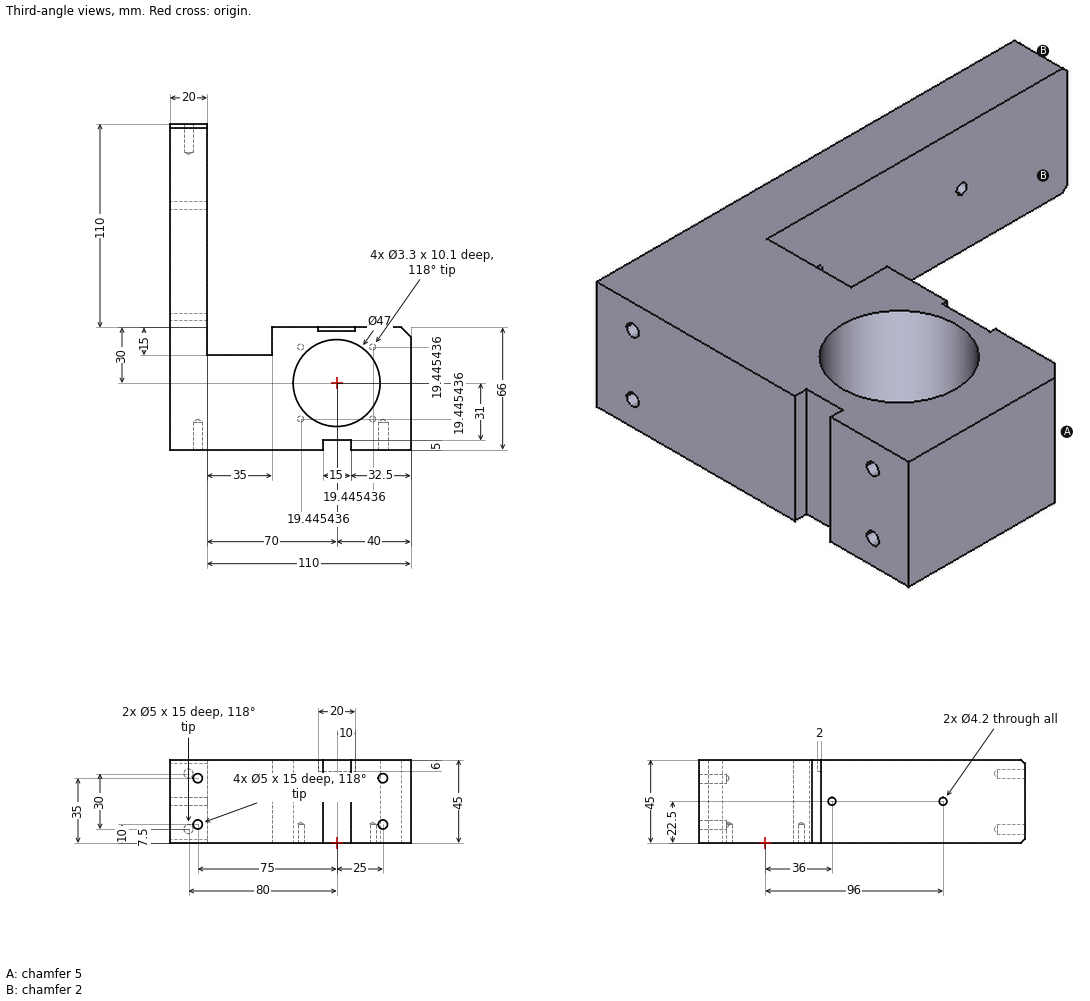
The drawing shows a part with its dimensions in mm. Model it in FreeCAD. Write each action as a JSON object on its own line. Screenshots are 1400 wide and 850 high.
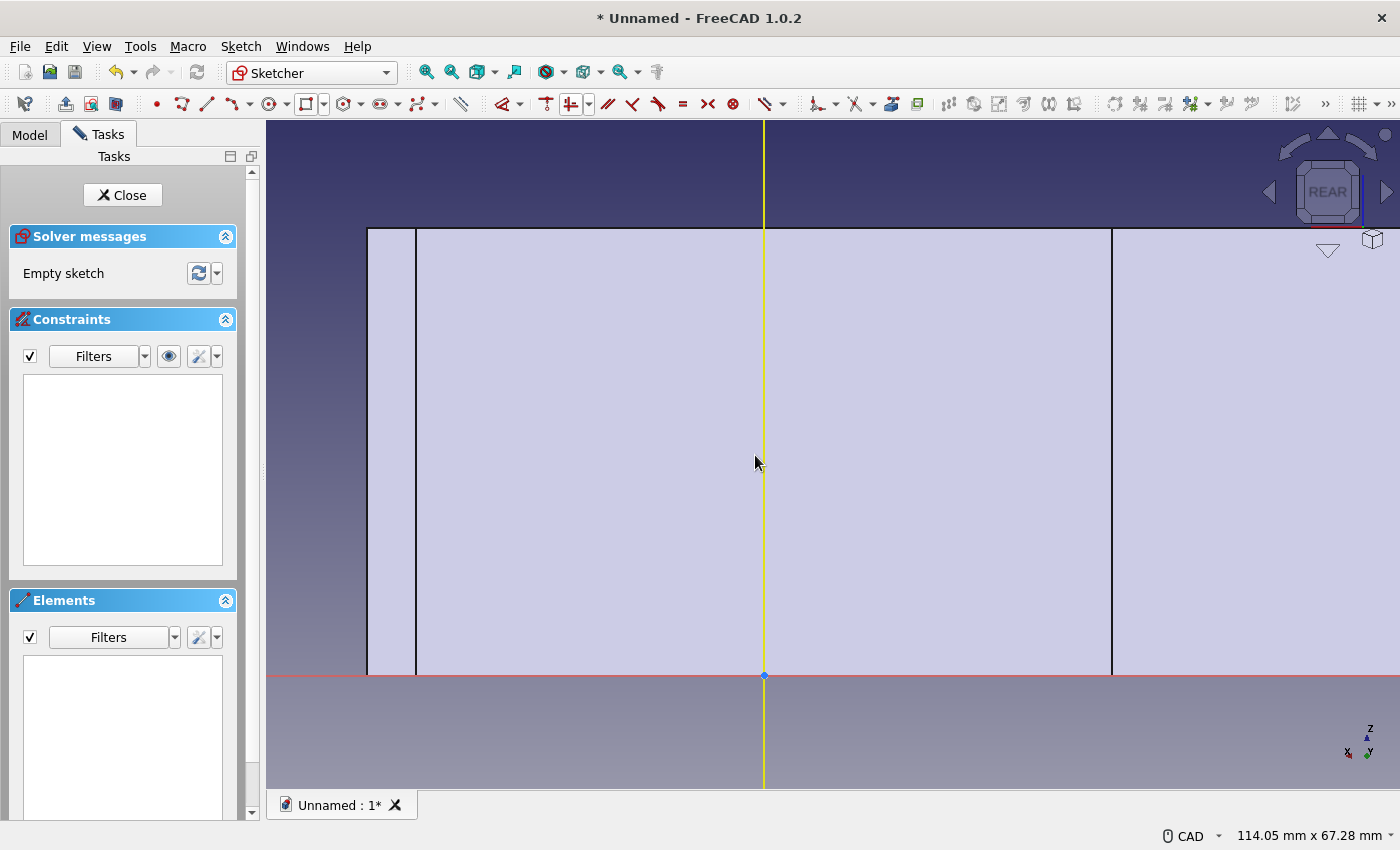
{"action": "left_click", "coordinate": [306, 104]}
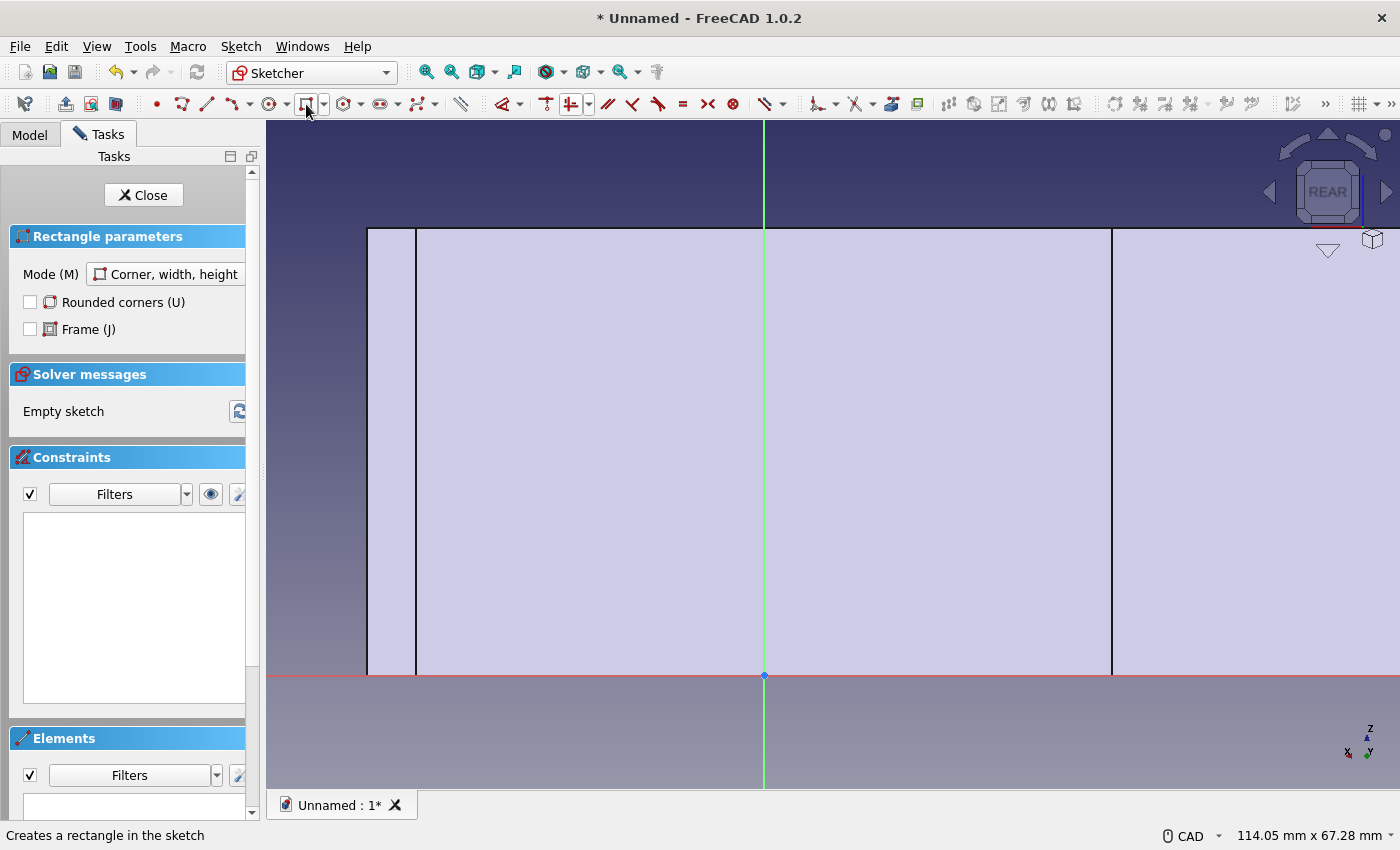
{"action": "left_click", "coordinate": [665, 228]}
{"action": "left_click", "coordinate": [864, 288]}
{"action": "key", "text": "Escape"}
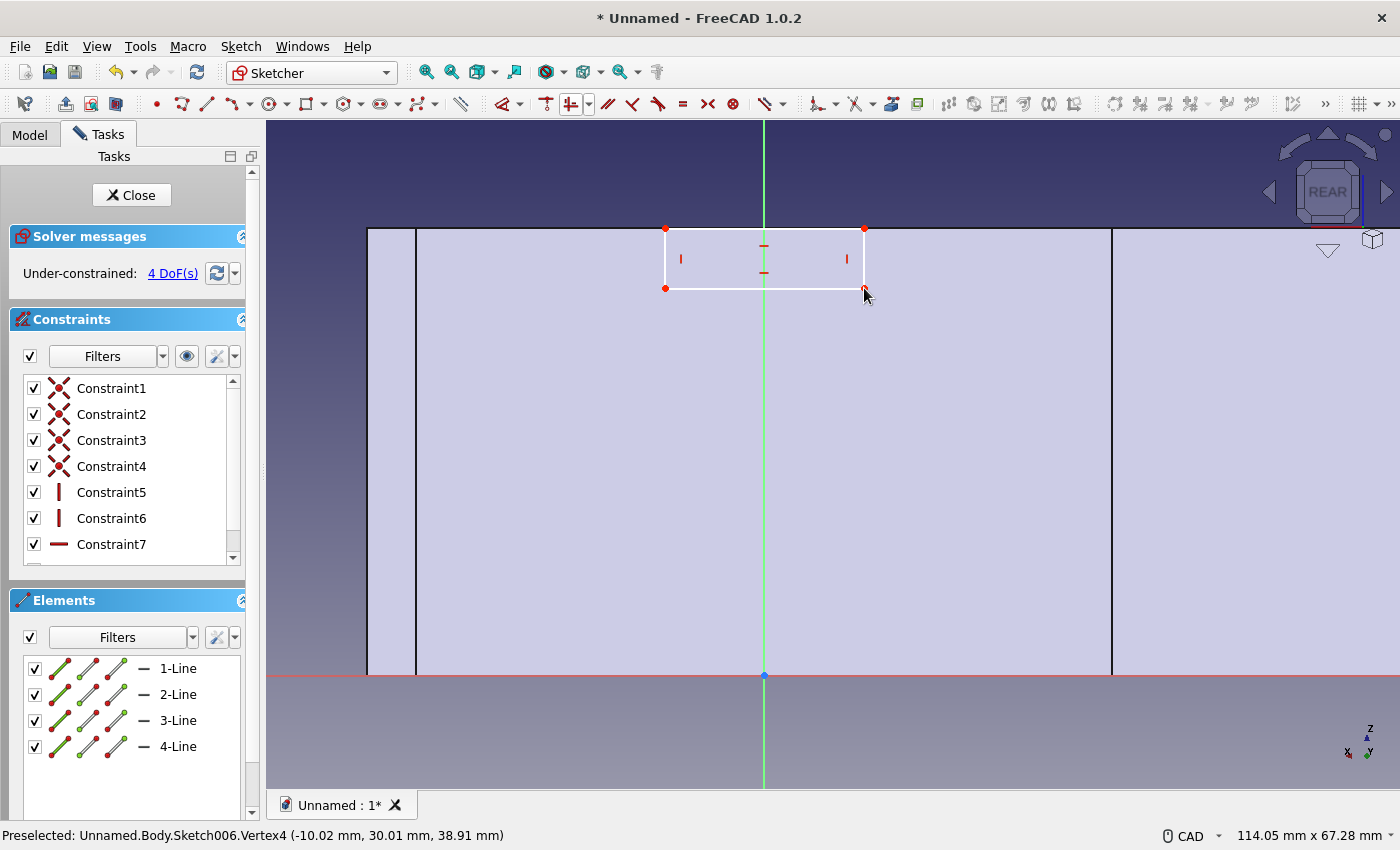
{"action": "left_click", "coordinate": [502, 104]}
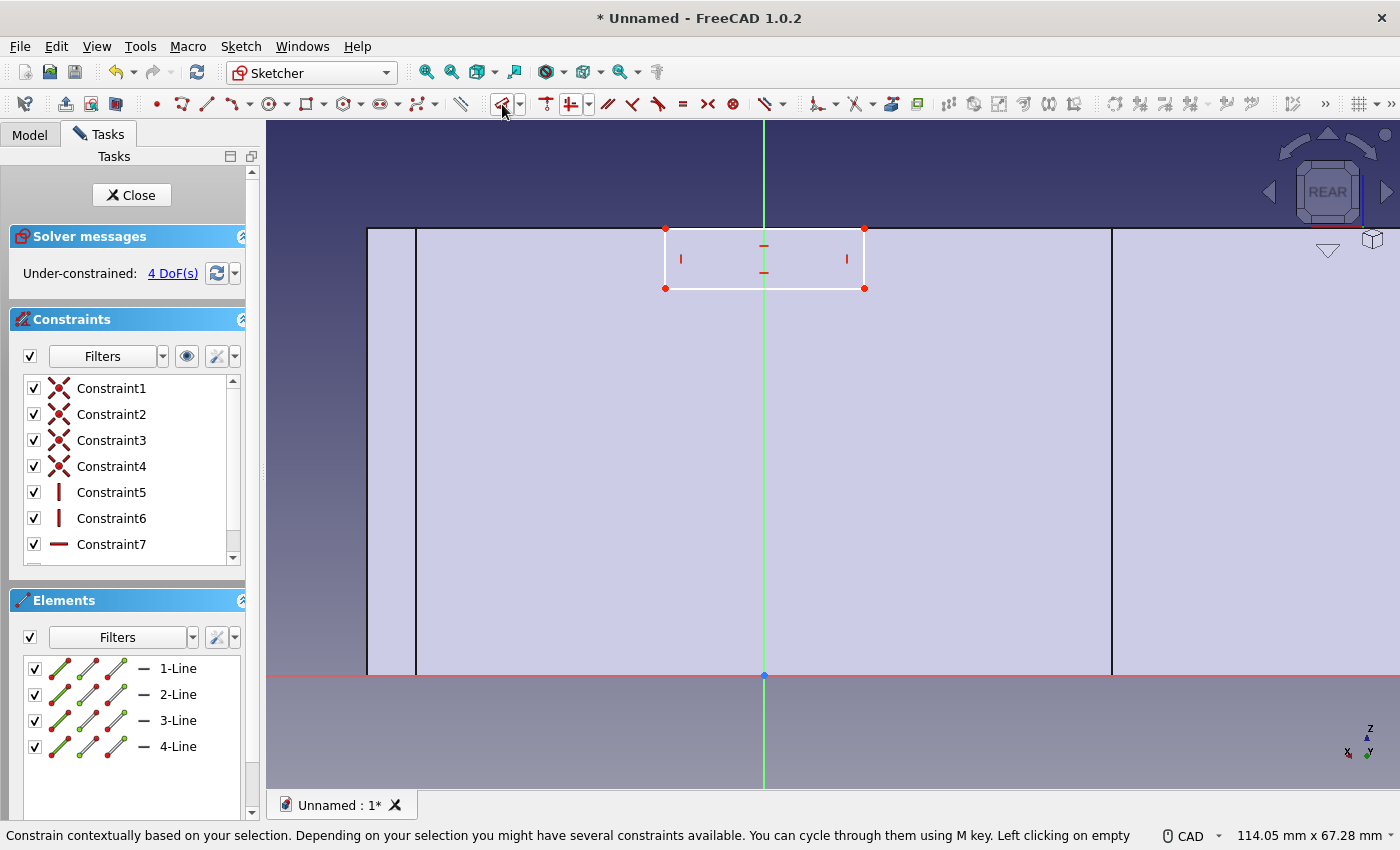
{"action": "left_click", "coordinate": [665, 247]}
{"action": "left_click", "coordinate": [631, 259]}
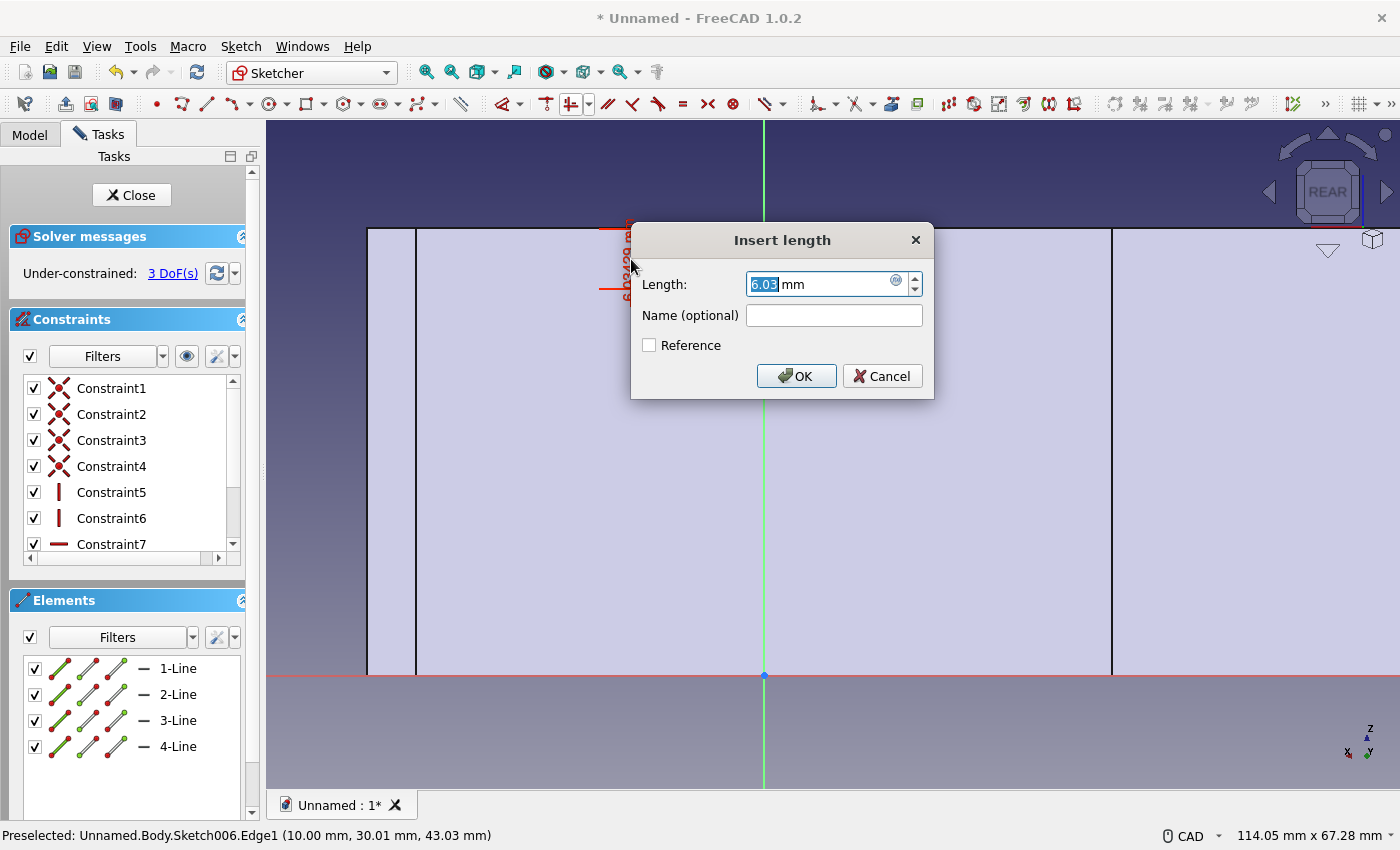
{"action": "type", "text": "6"}
{"action": "key", "text": "Return"}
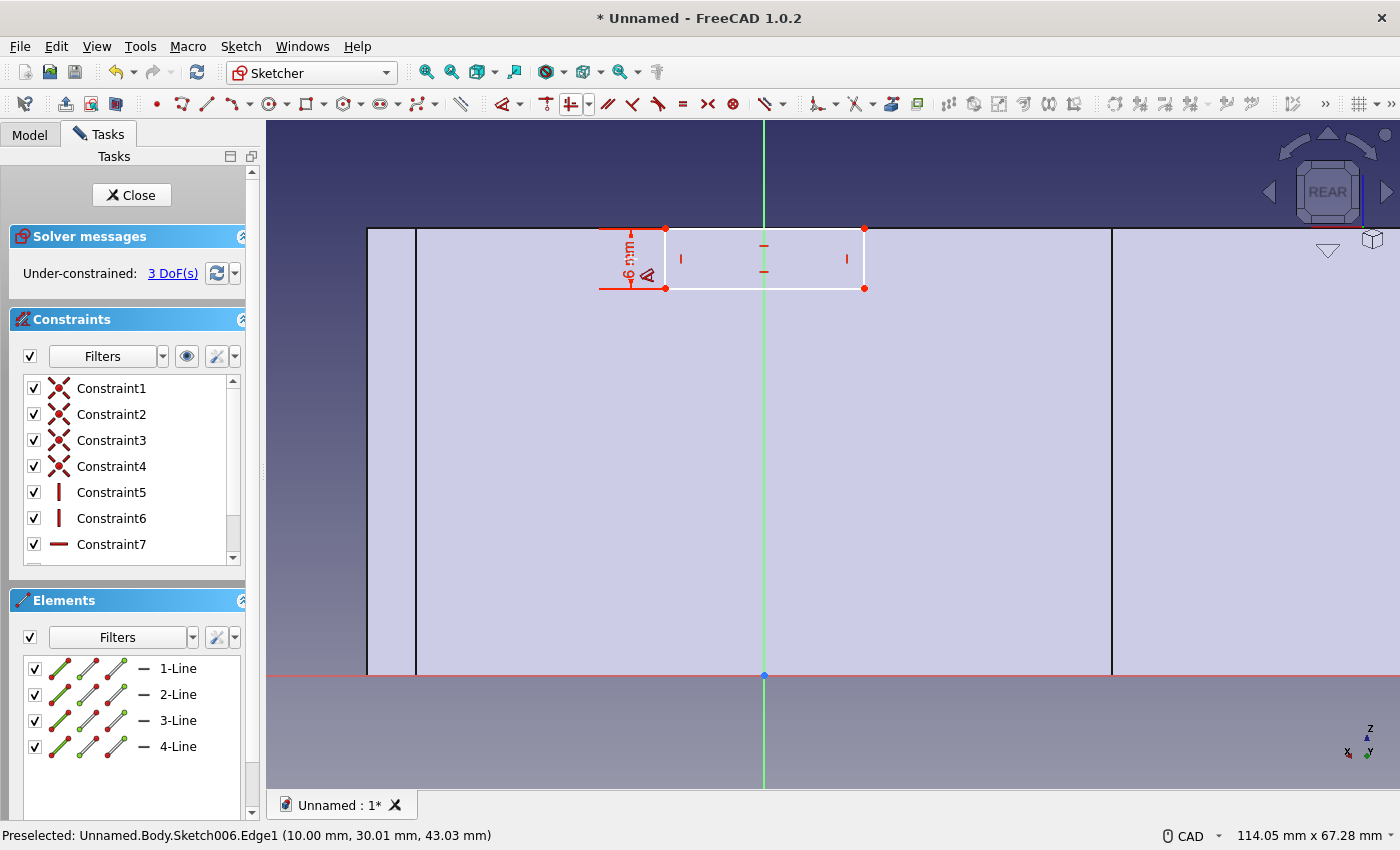
{"action": "left_click", "coordinate": [725, 289]}
{"action": "left_click", "coordinate": [719, 255]}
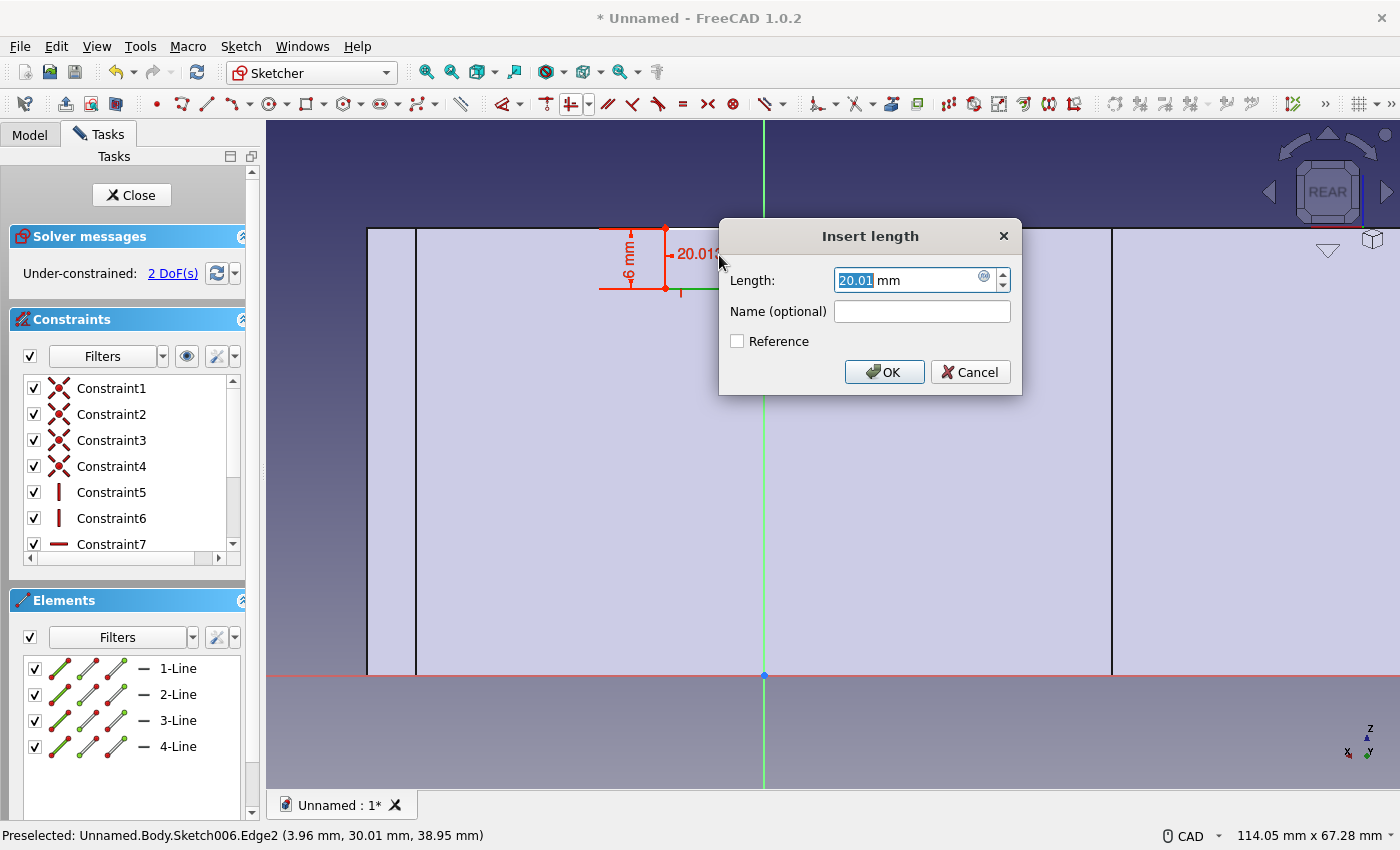
{"action": "type", "text": "20"}
{"action": "key", "text": "Return"}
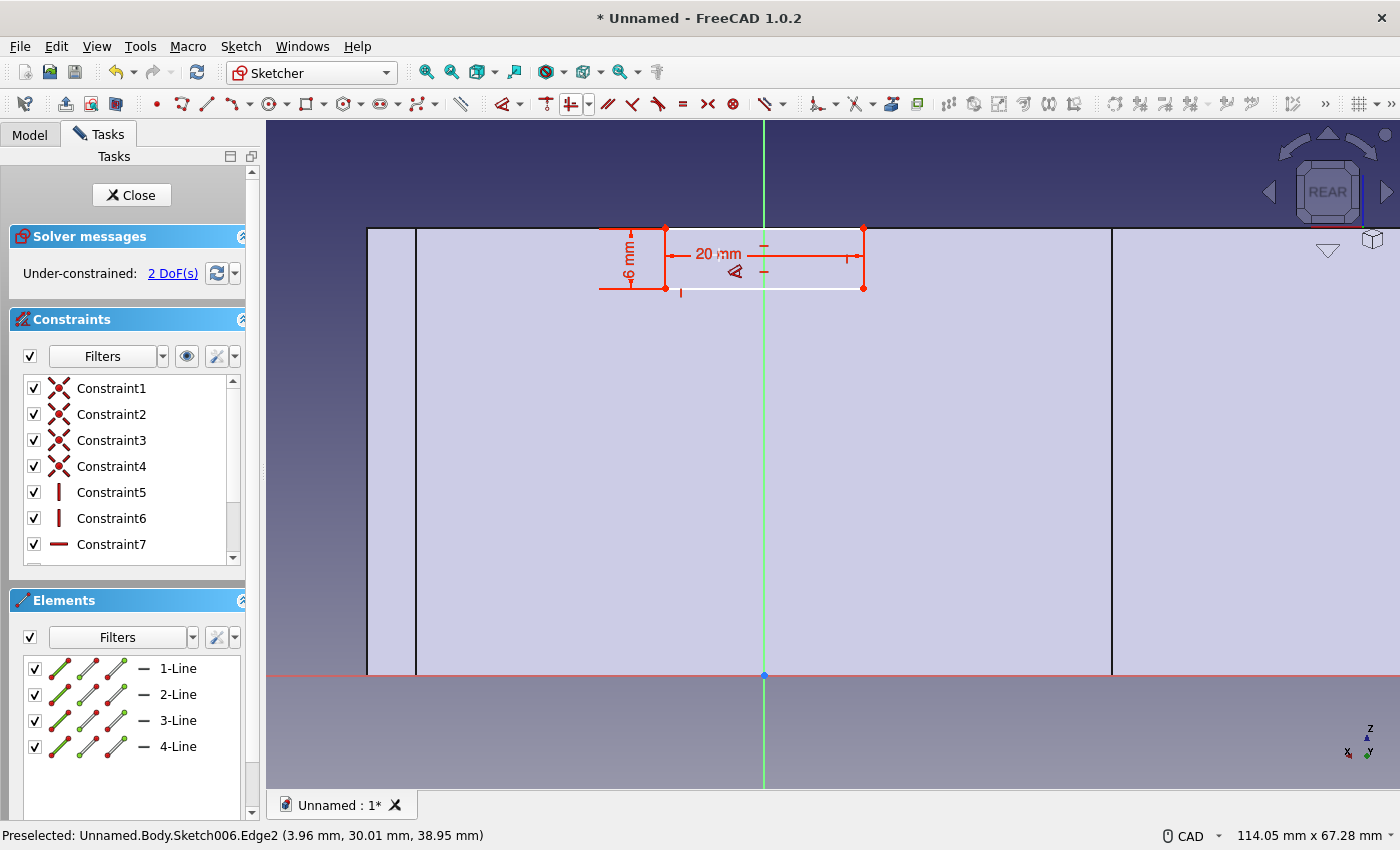
{"action": "left_click", "coordinate": [665, 229]}
{"action": "left_click", "coordinate": [715, 710]}